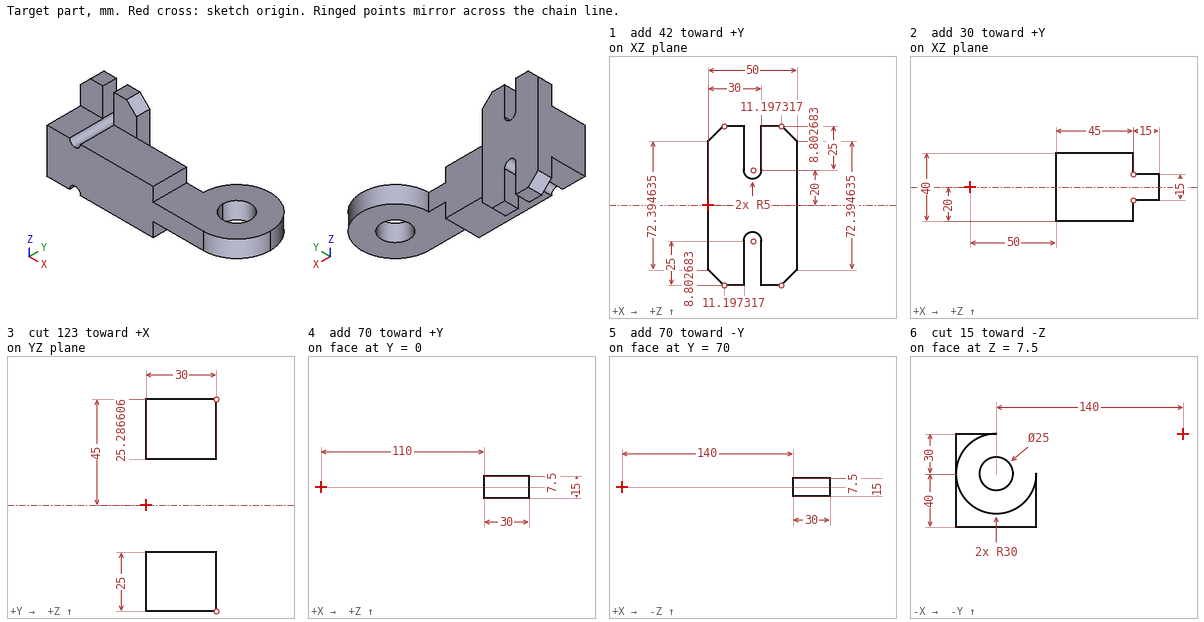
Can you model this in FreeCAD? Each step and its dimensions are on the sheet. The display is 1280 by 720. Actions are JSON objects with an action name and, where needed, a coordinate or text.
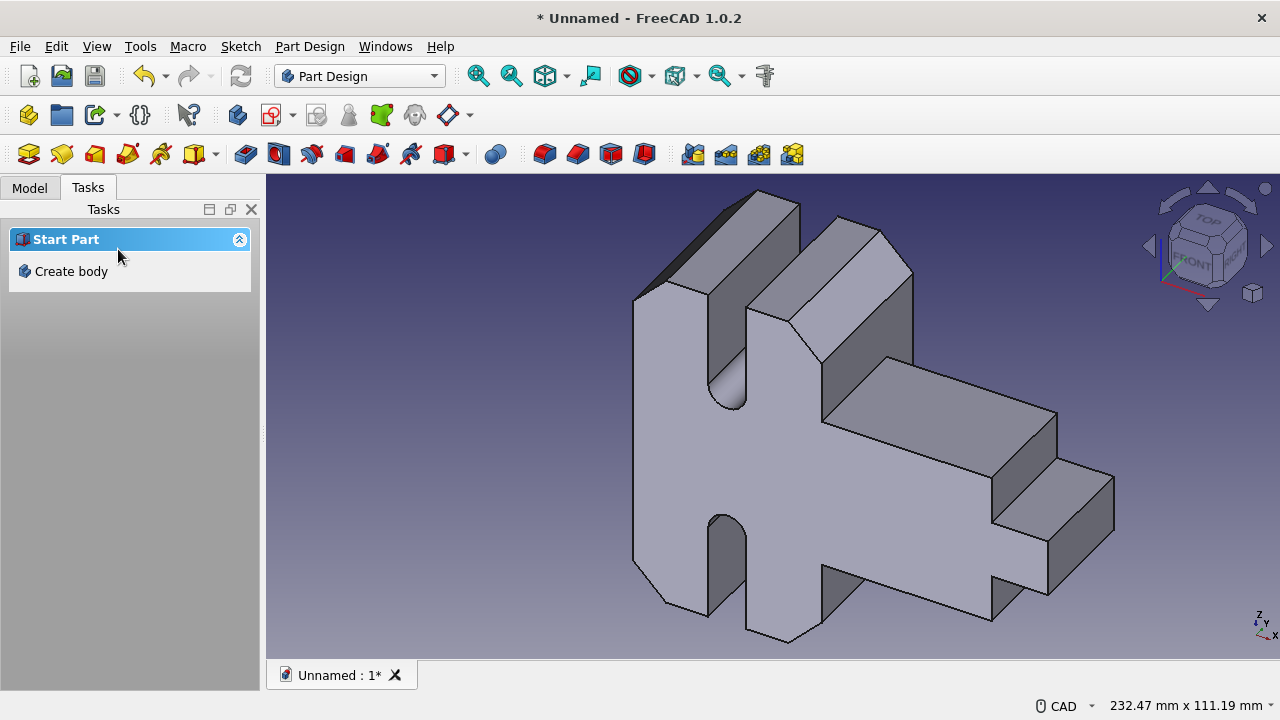
{"action": "key", "text": "v f"}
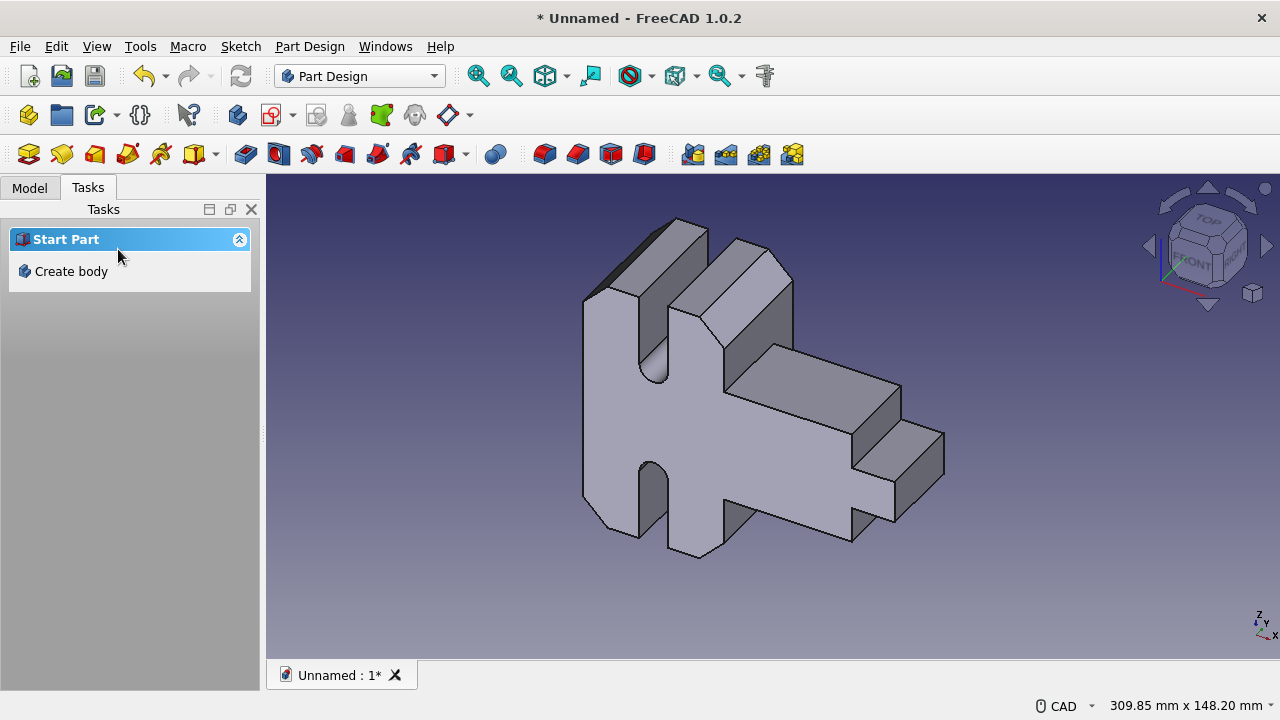
{"action": "left_click", "coordinate": [270, 116]}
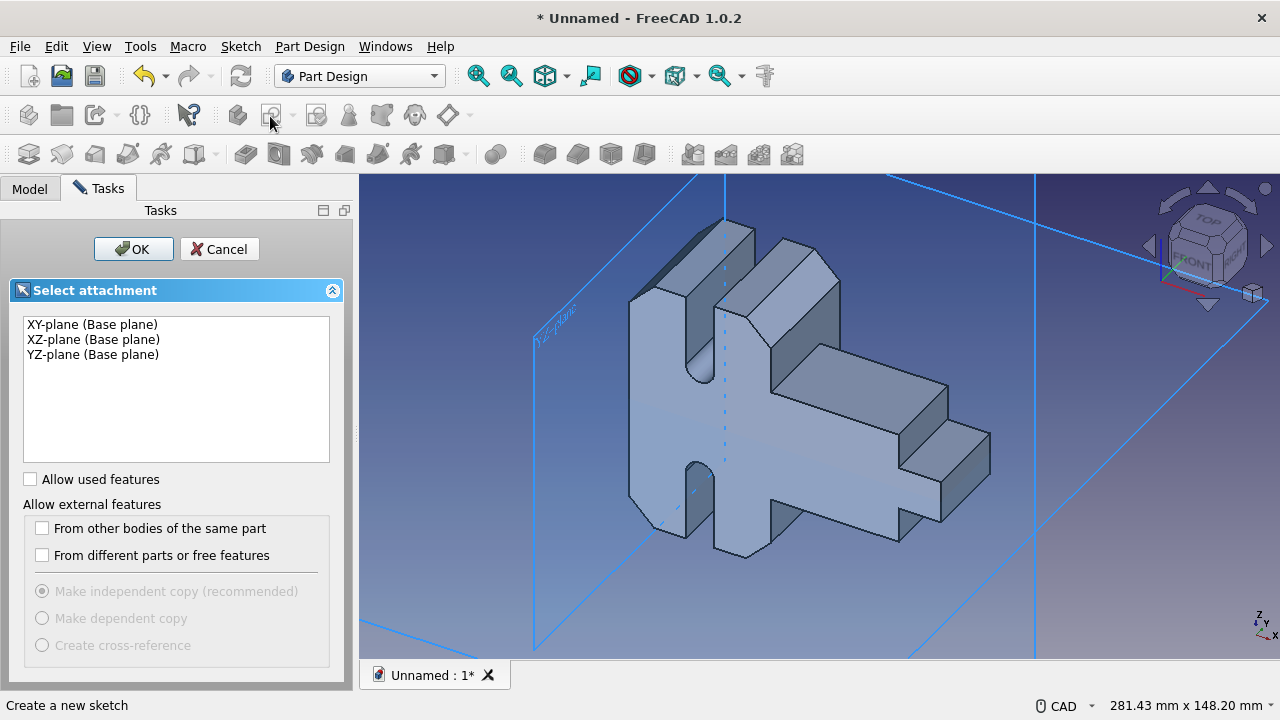
{"action": "left_click", "coordinate": [84, 354]}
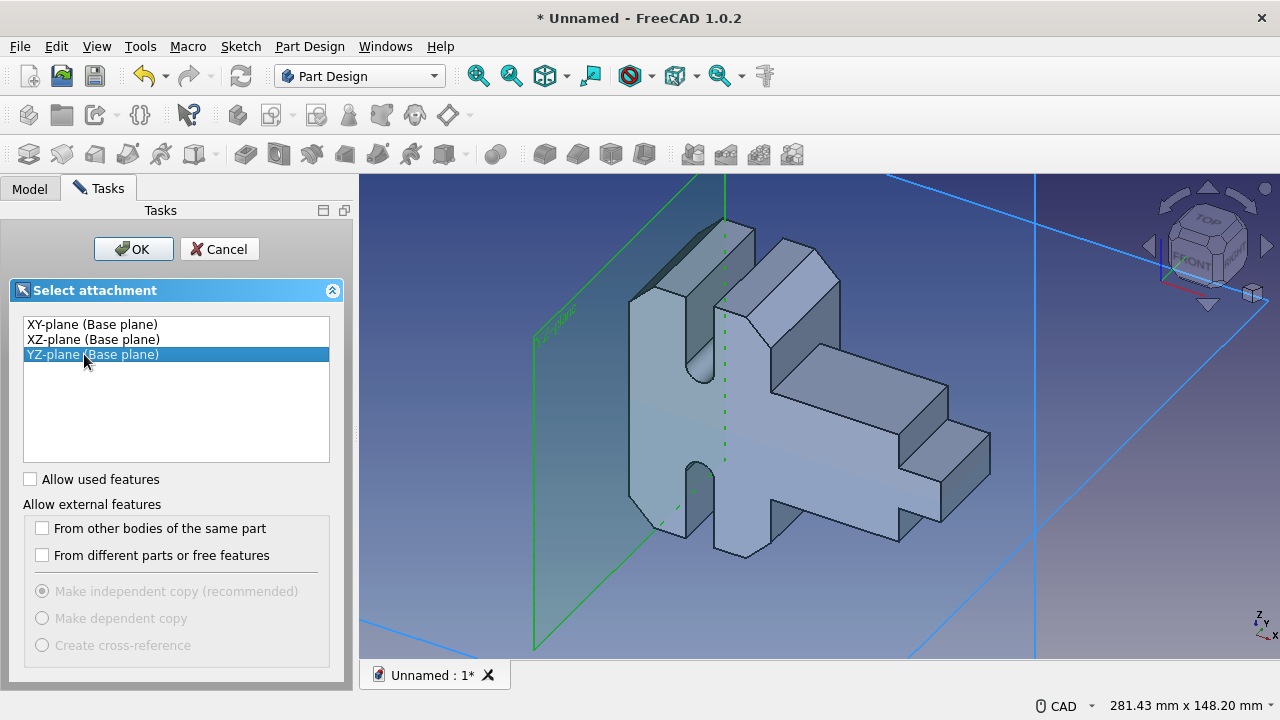
{"action": "left_click", "coordinate": [134, 249]}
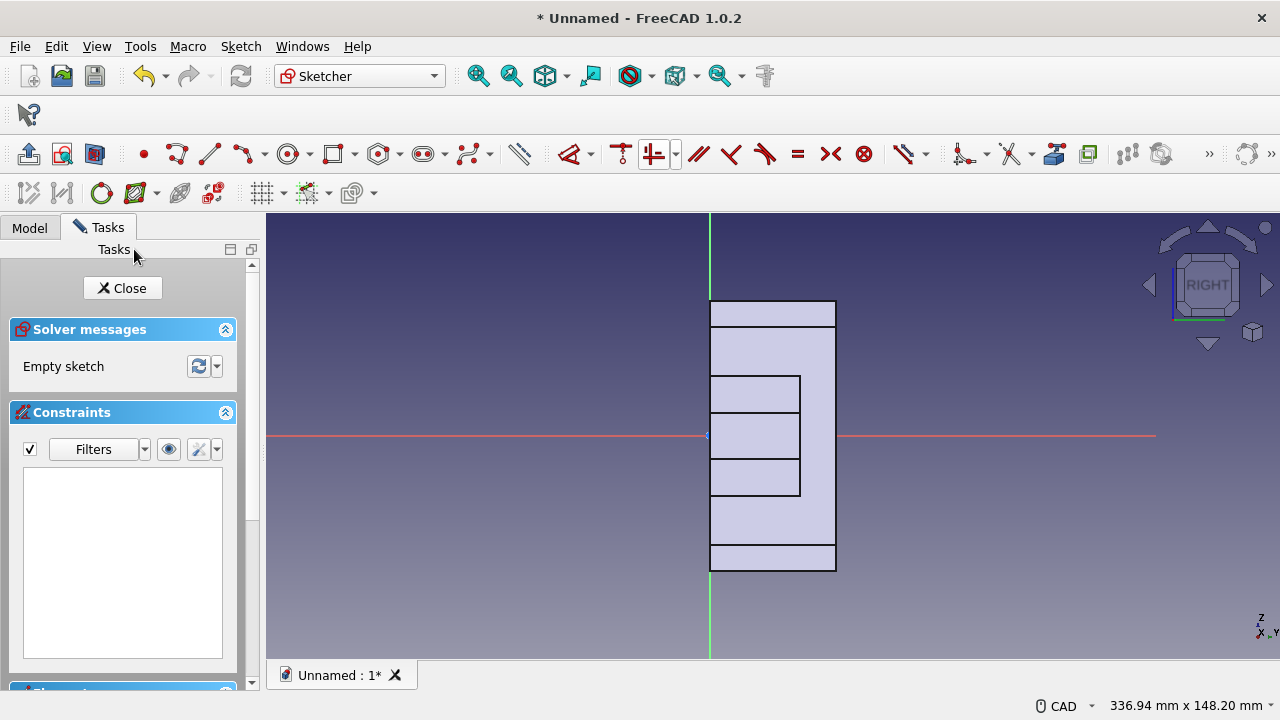
{"action": "left_click", "coordinate": [95, 154]}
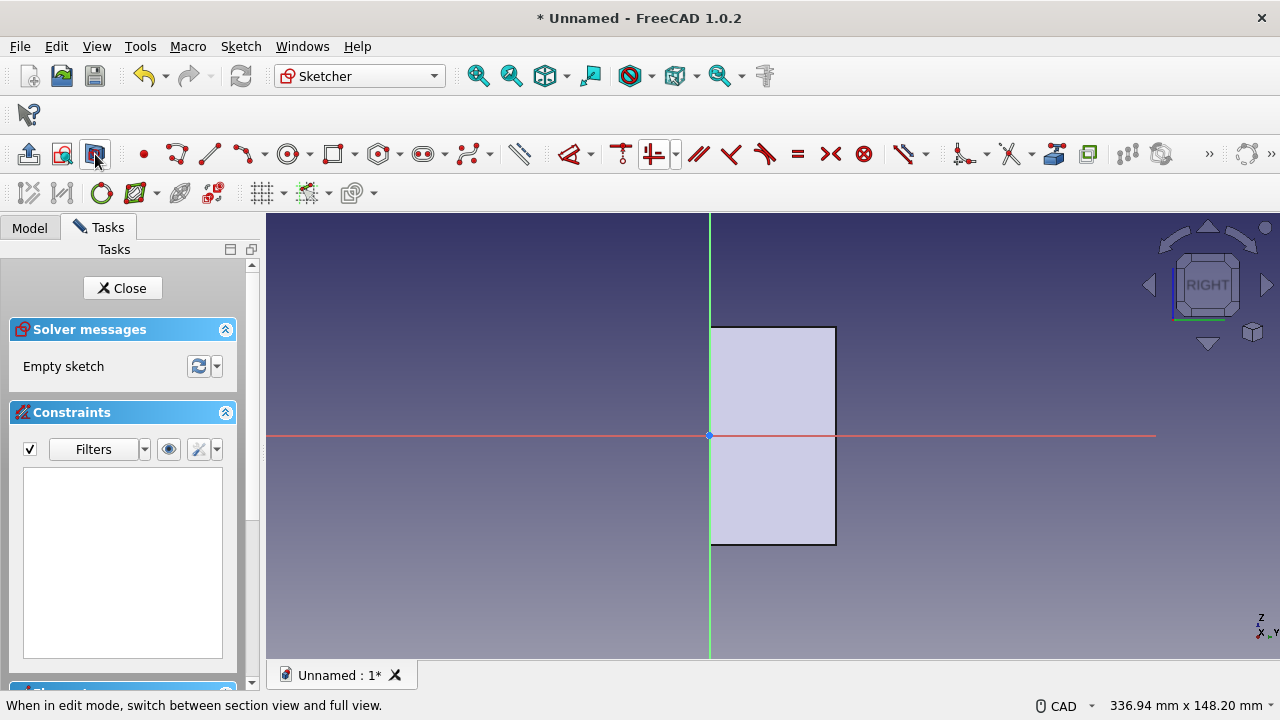
{"action": "left_click", "coordinate": [332, 154]}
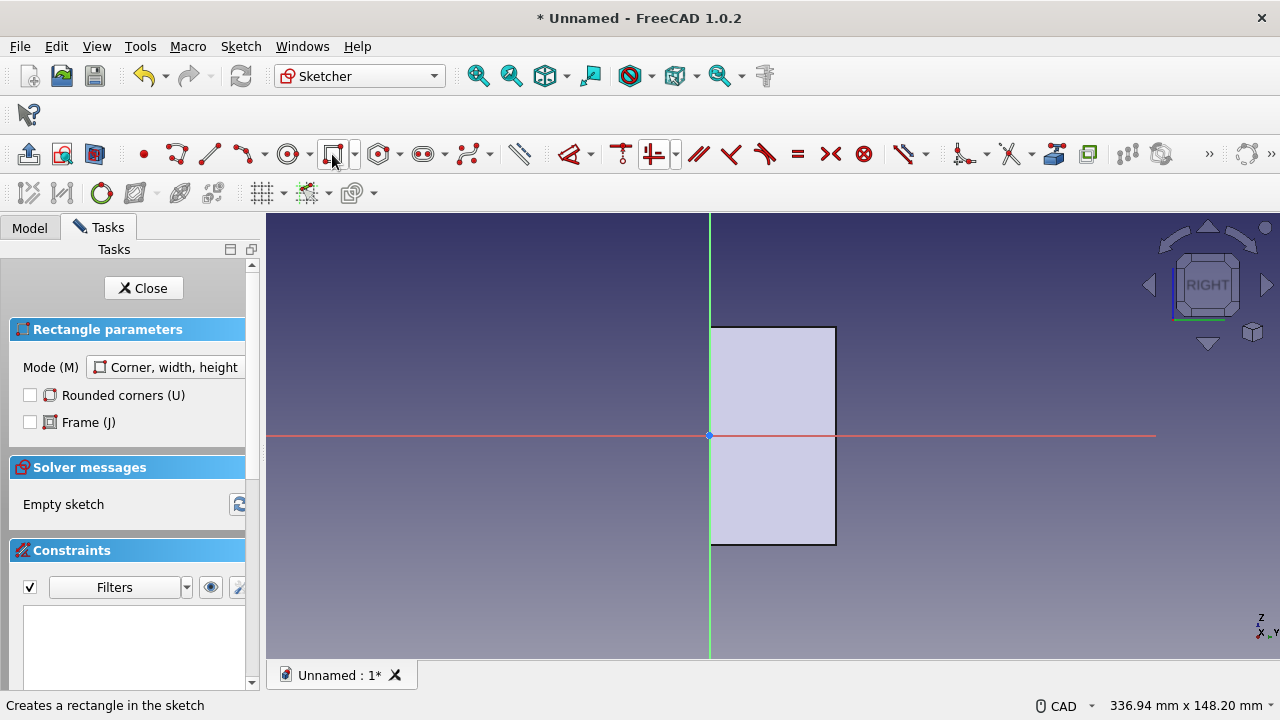
{"action": "left_click", "coordinate": [710, 301]}
{"action": "left_click", "coordinate": [800, 377]}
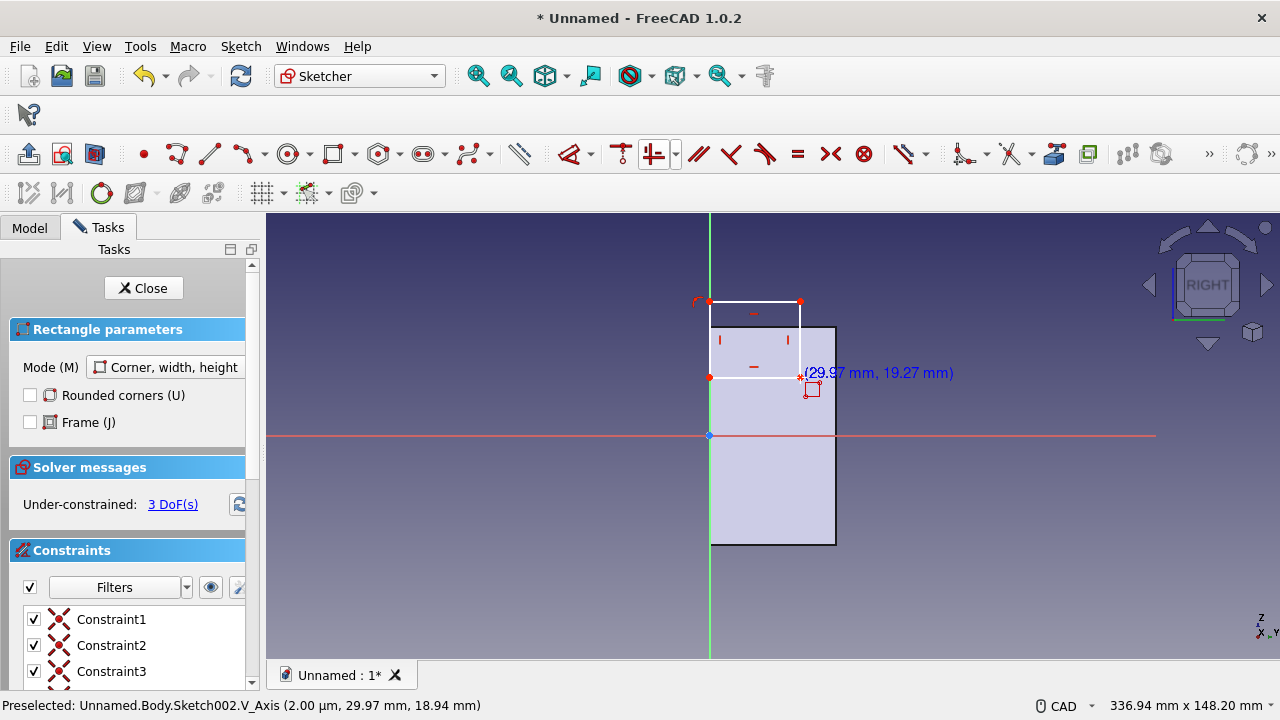
{"action": "left_click", "coordinate": [710, 496]}
{"action": "left_click", "coordinate": [800, 571]}
{"action": "key", "text": "Escape"}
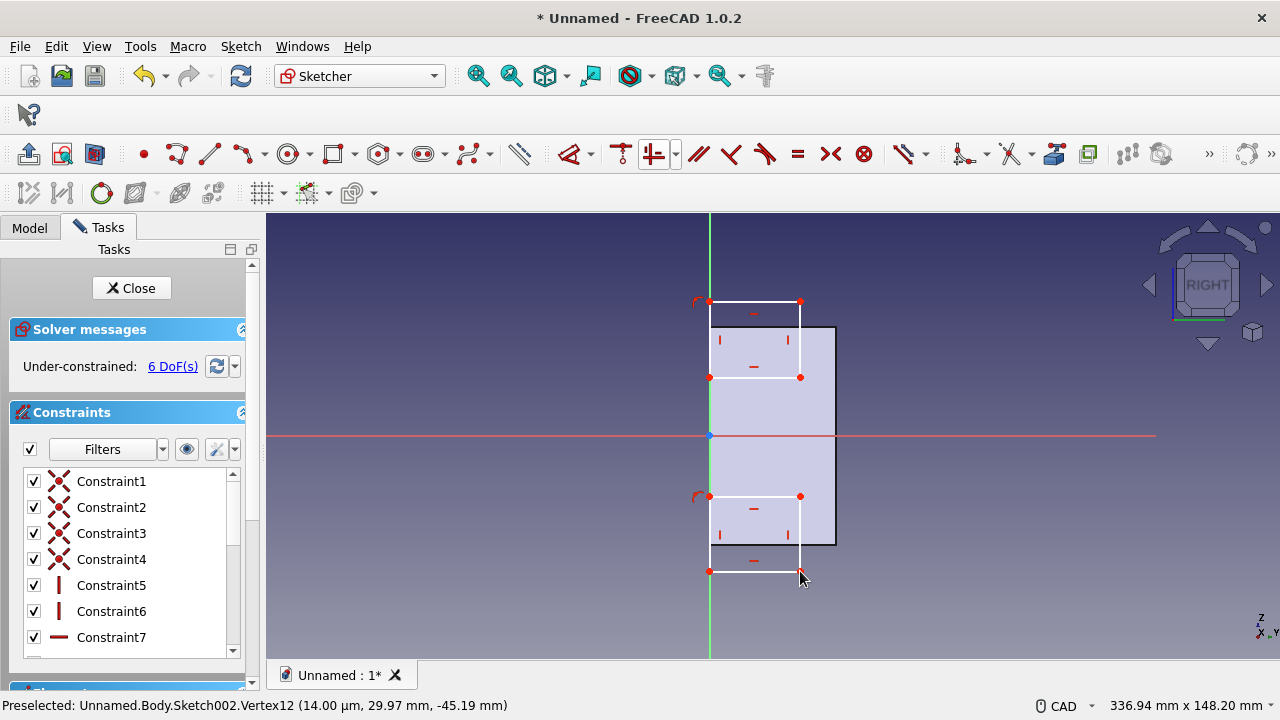
{"action": "left_click", "coordinate": [800, 302]}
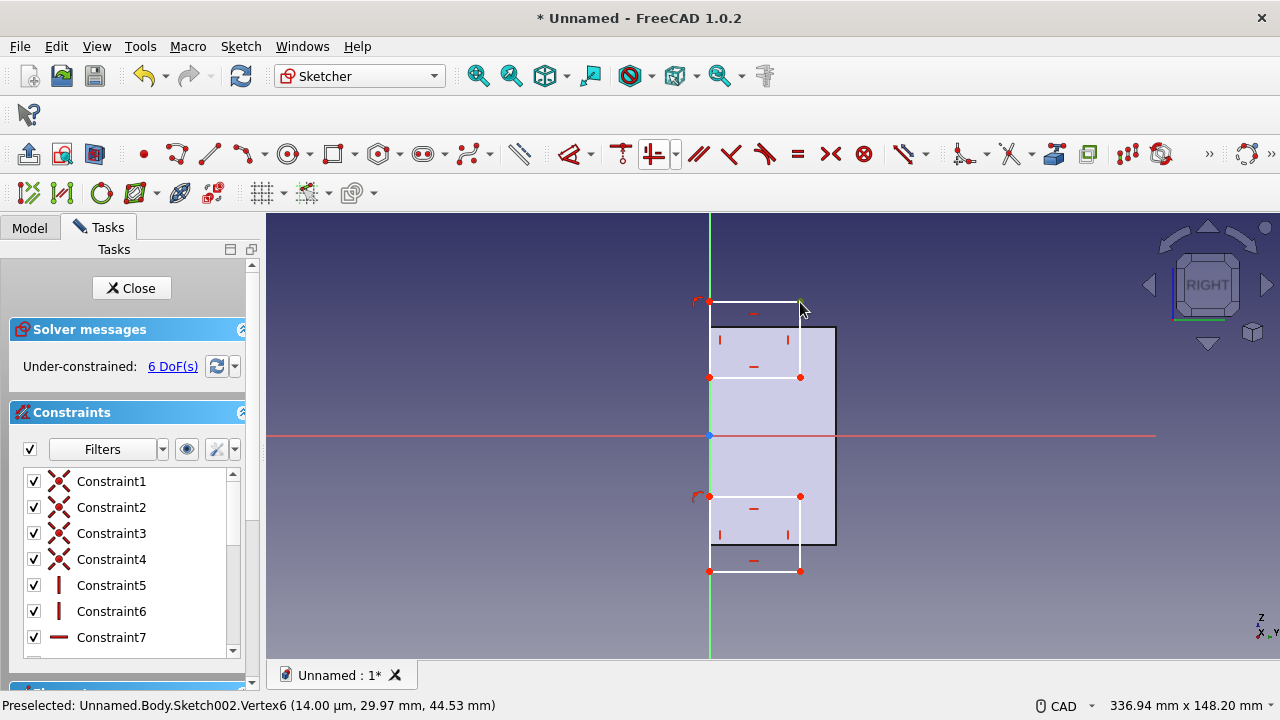
{"action": "left_click", "coordinate": [800, 572]}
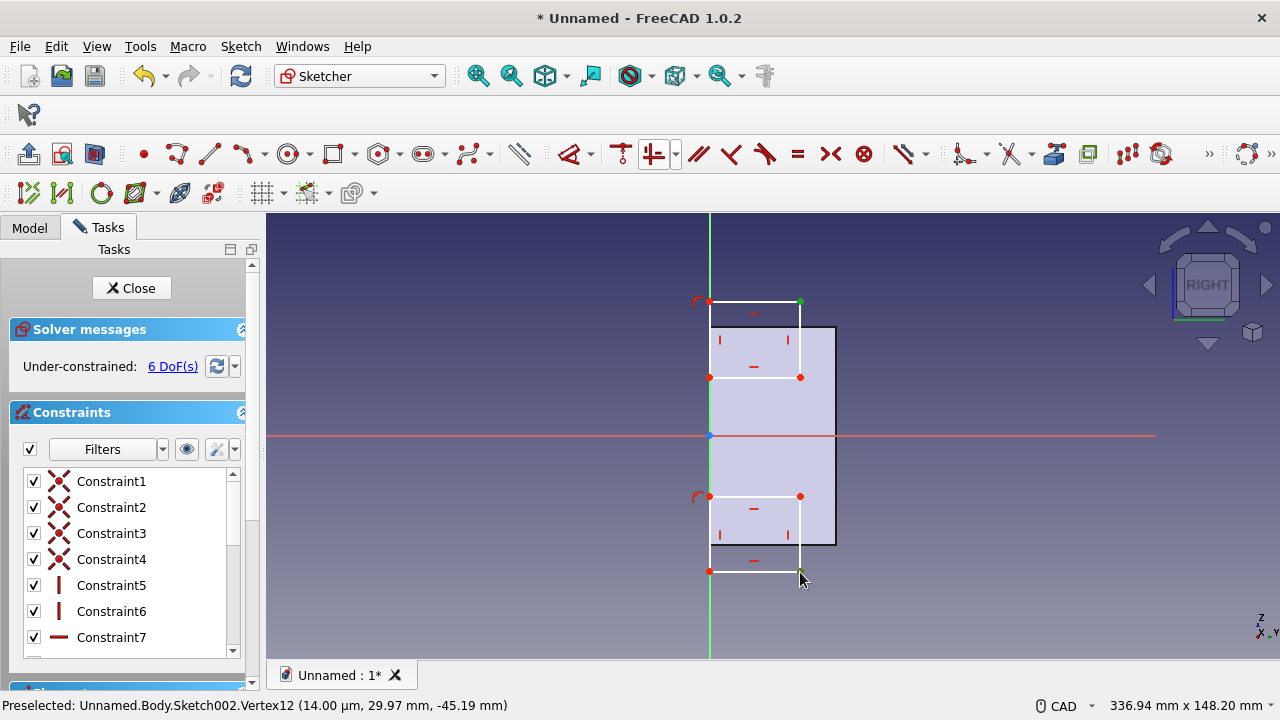
{"action": "left_click", "coordinate": [353, 436]}